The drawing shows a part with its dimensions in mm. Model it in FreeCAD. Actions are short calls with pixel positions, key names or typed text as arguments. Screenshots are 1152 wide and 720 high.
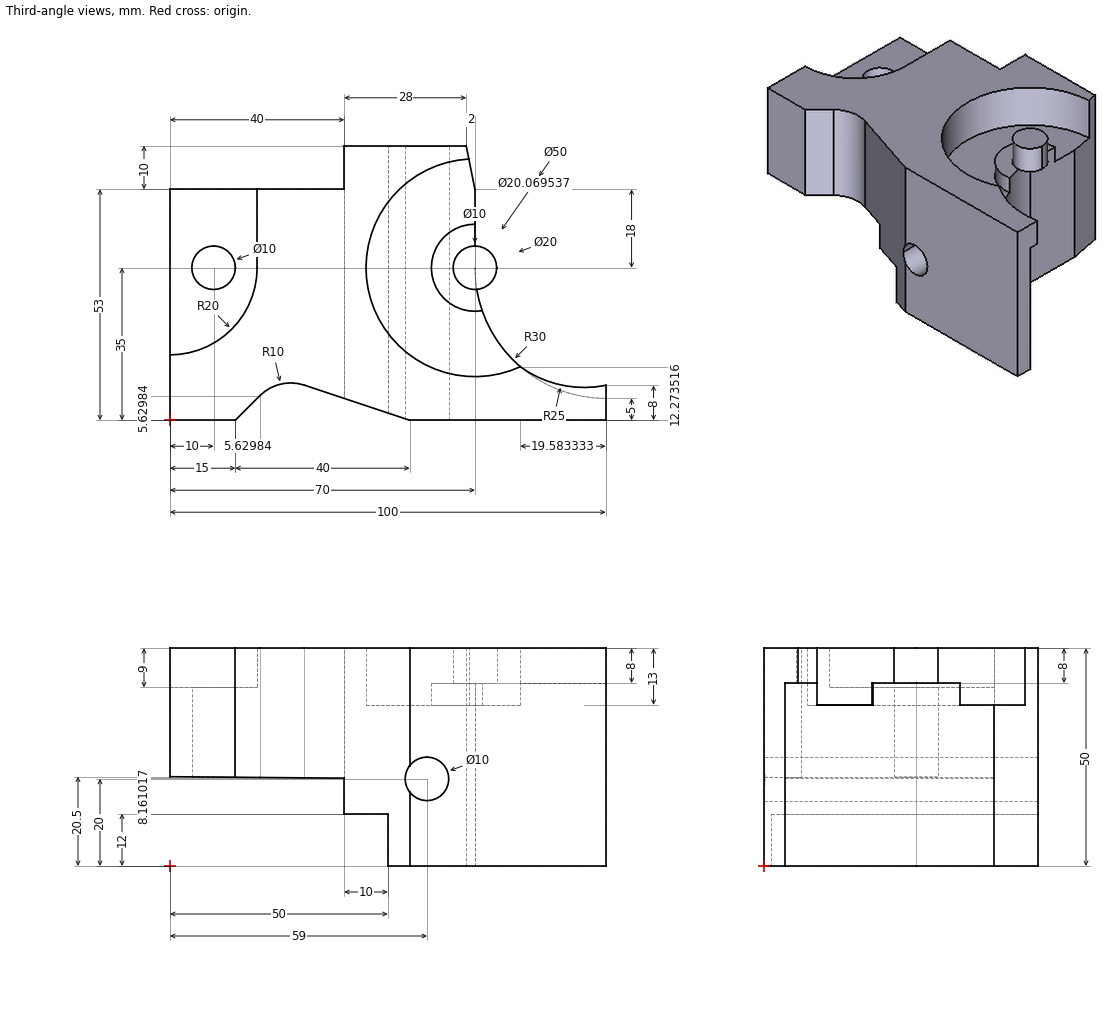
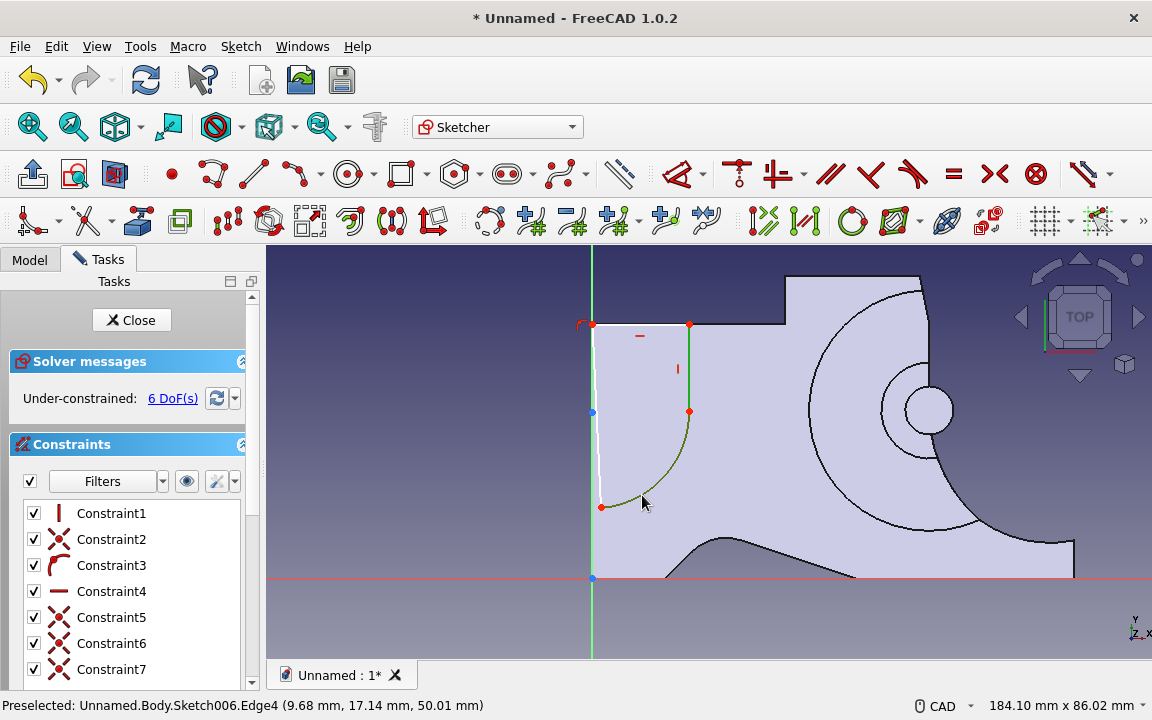
click(913, 174)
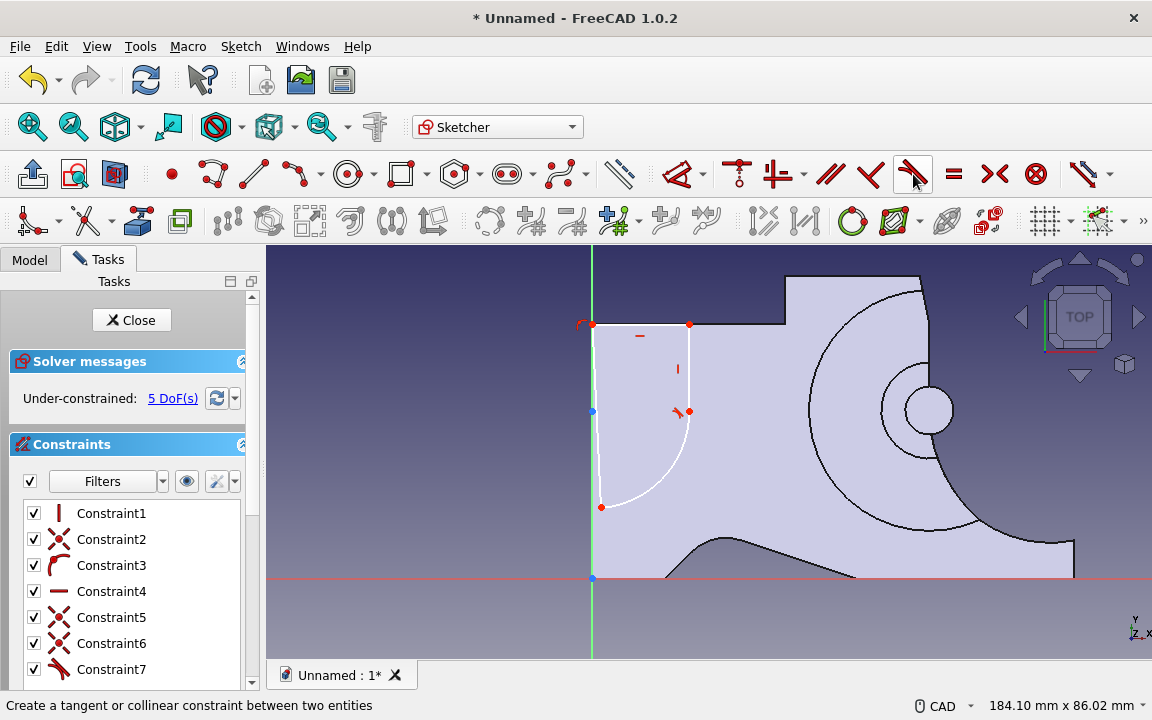
click(595, 380)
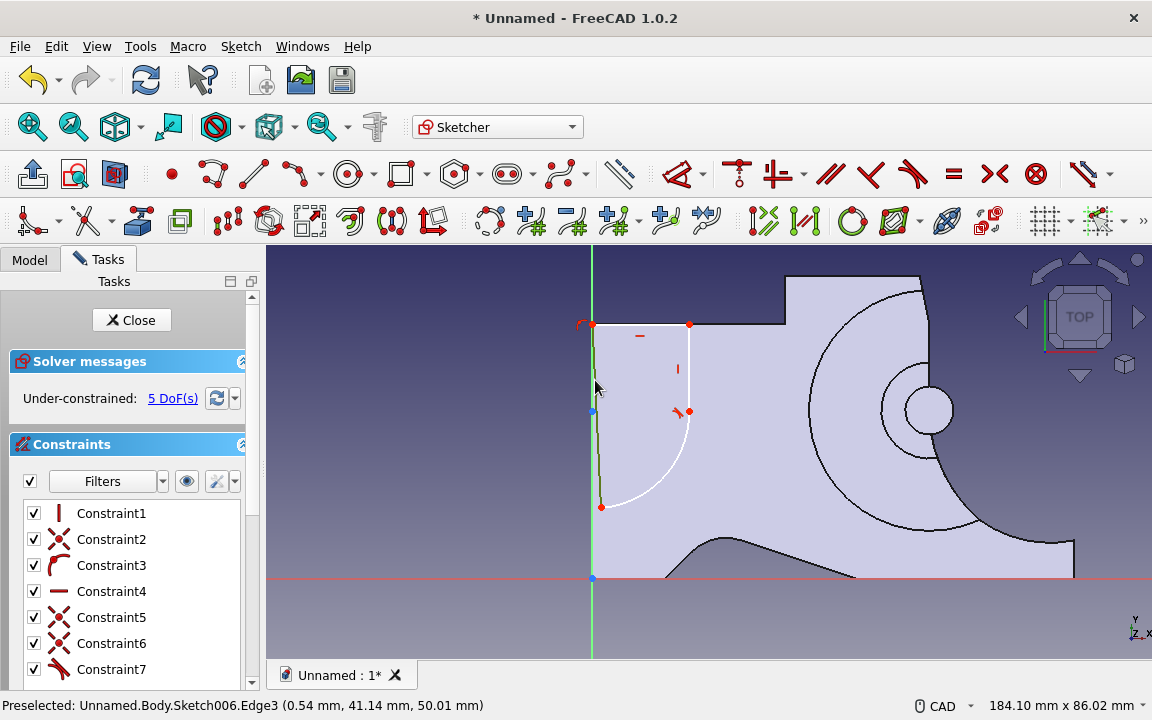
key(v)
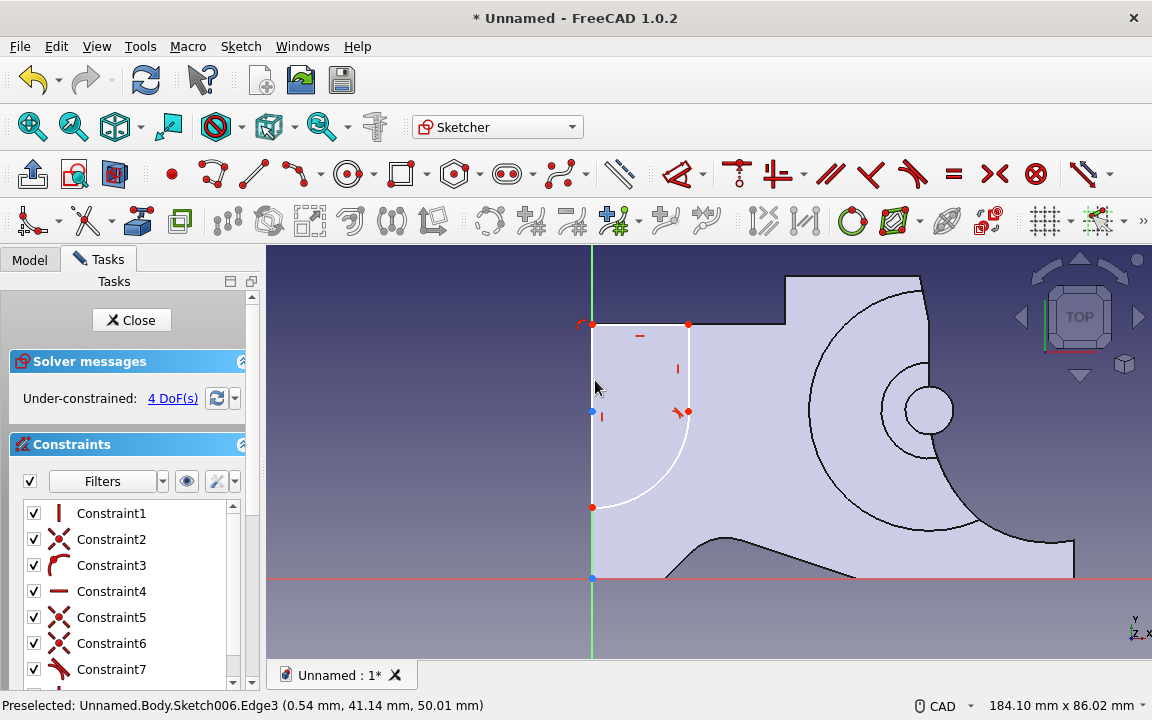
click(593, 412)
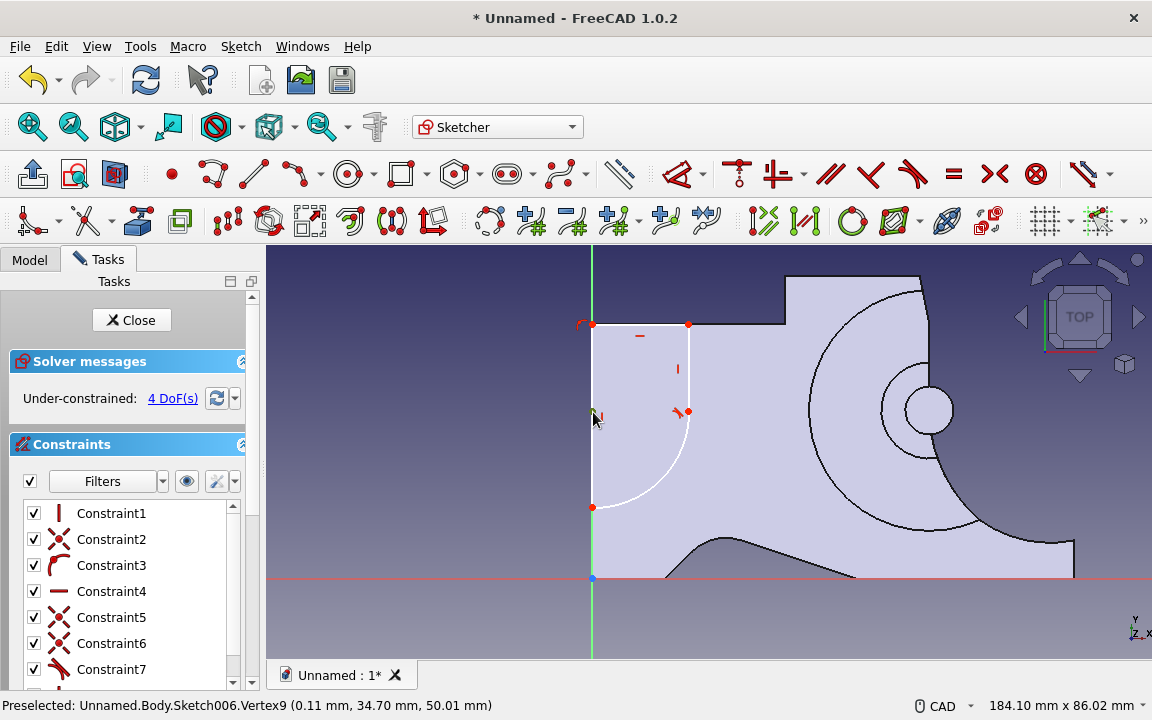
click(592, 605)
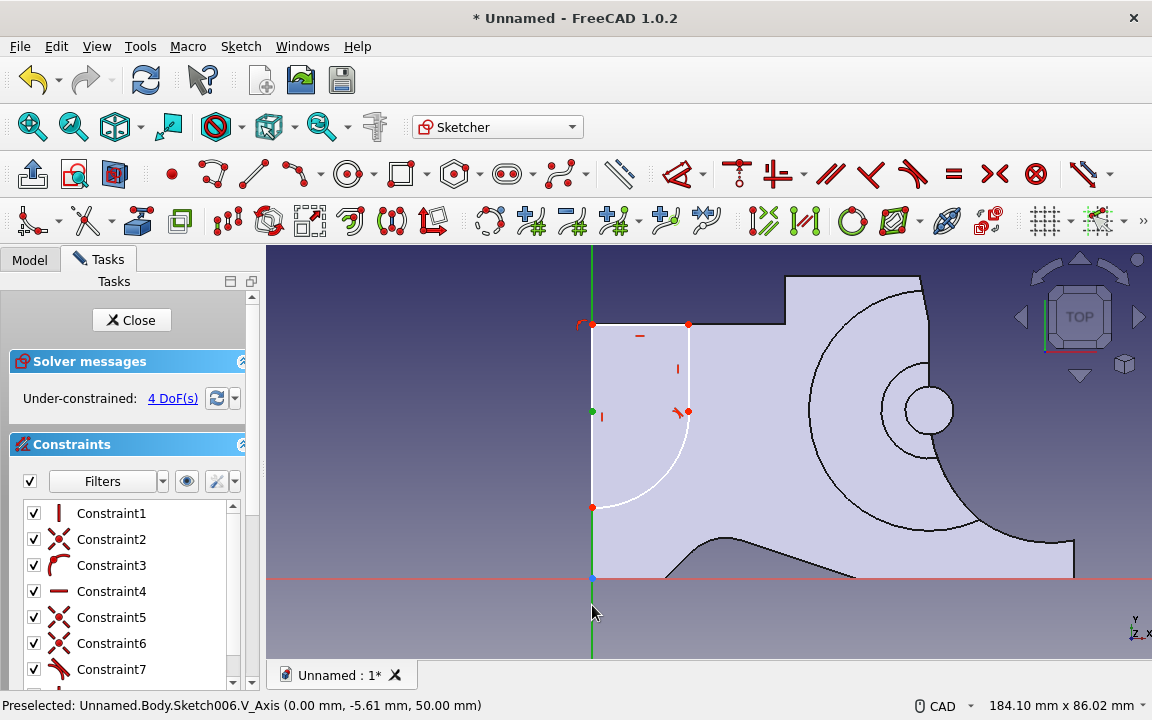
click(737, 174)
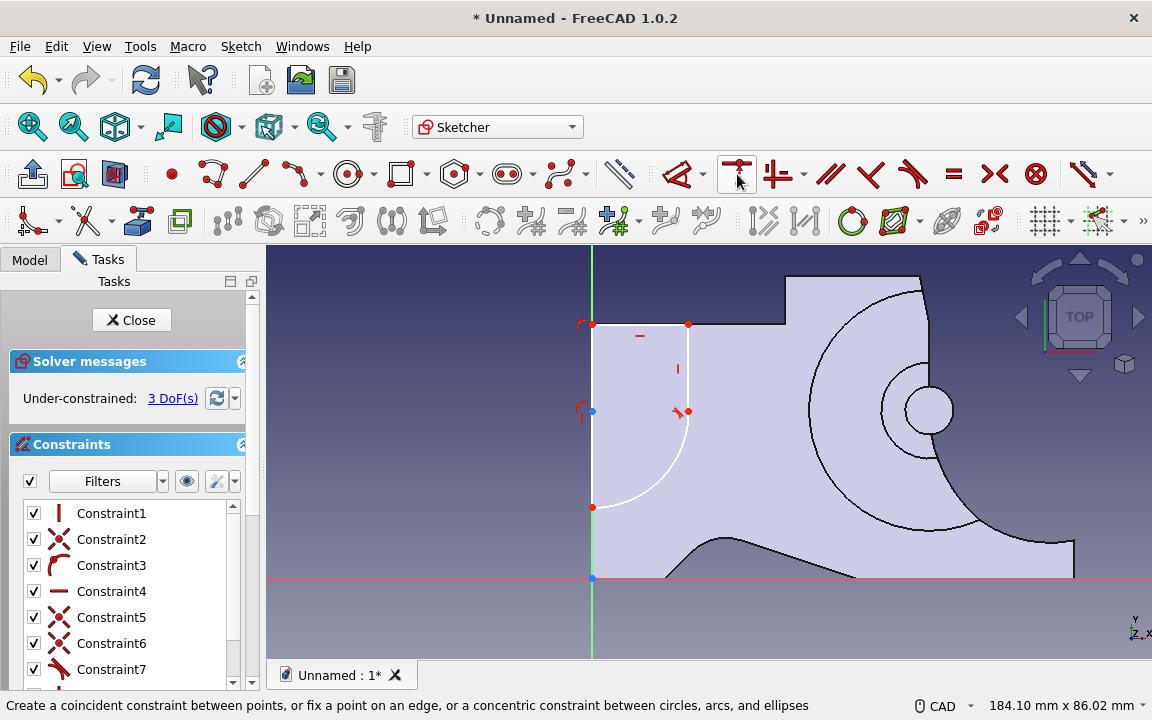
key(d)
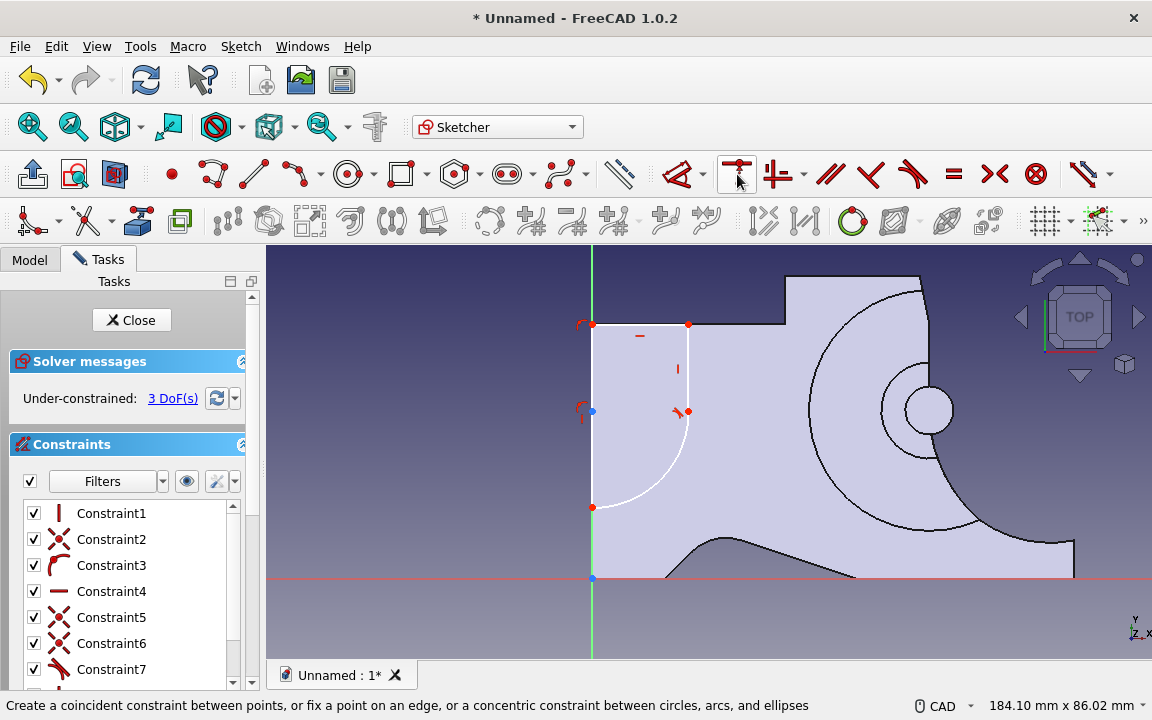
click(636, 498)
click(650, 527)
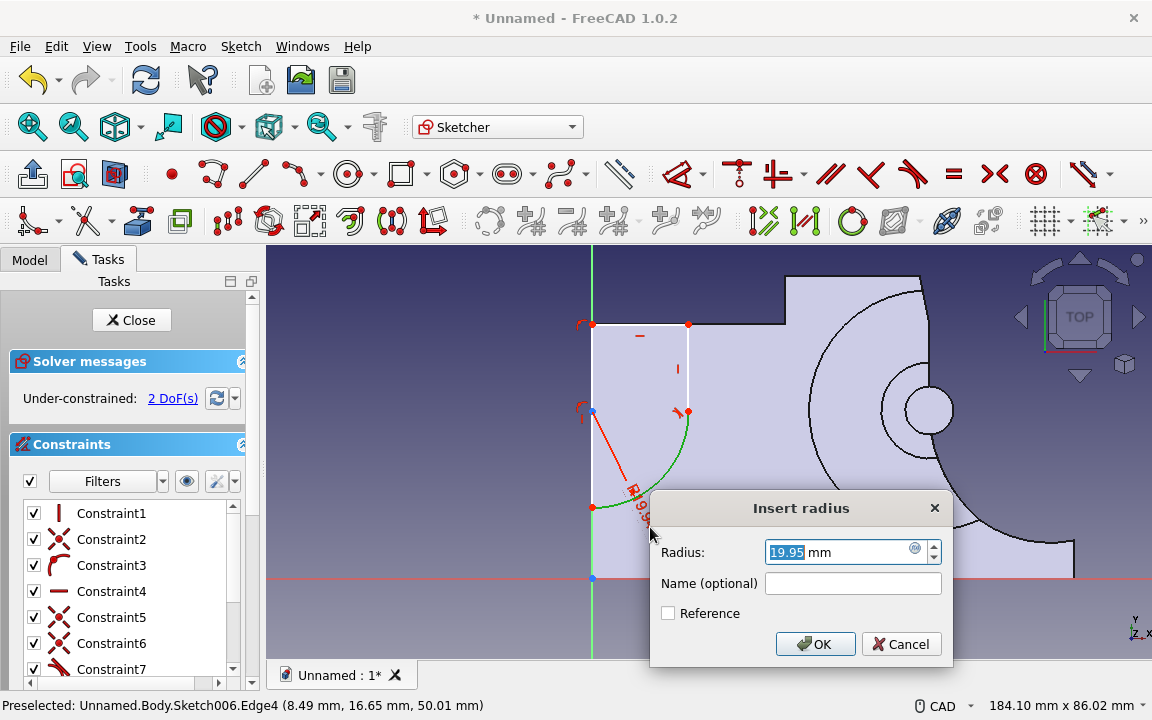
text(20)
key(Return)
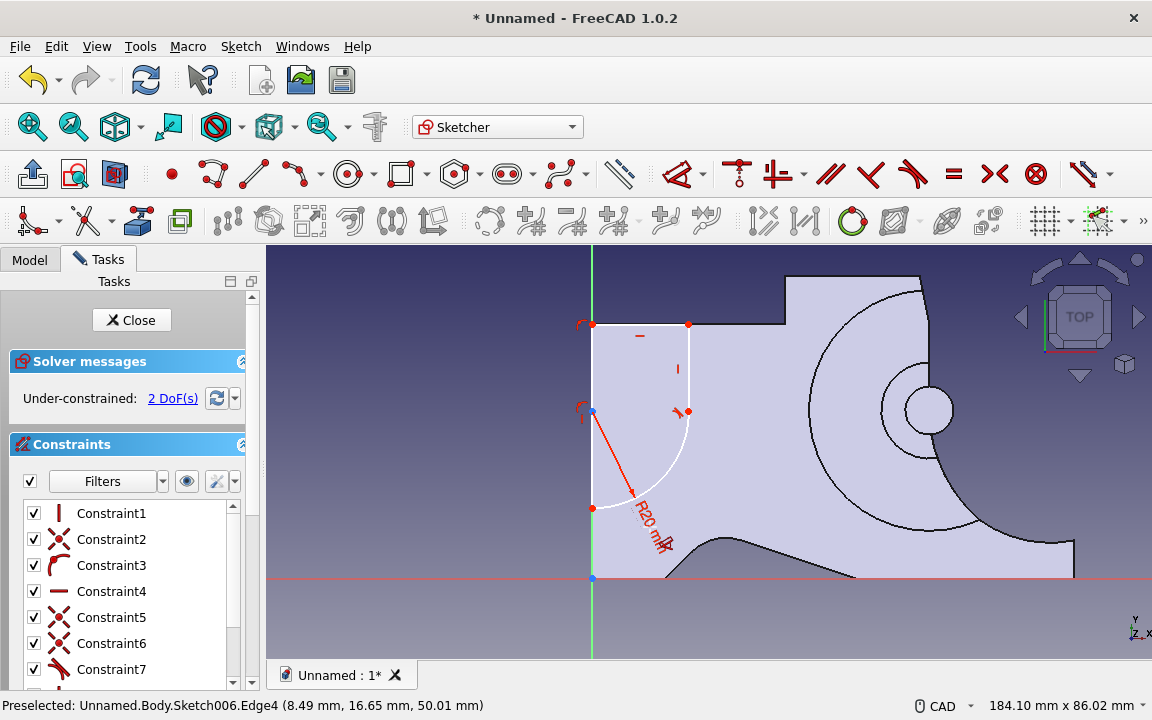
click(689, 386)
click(723, 369)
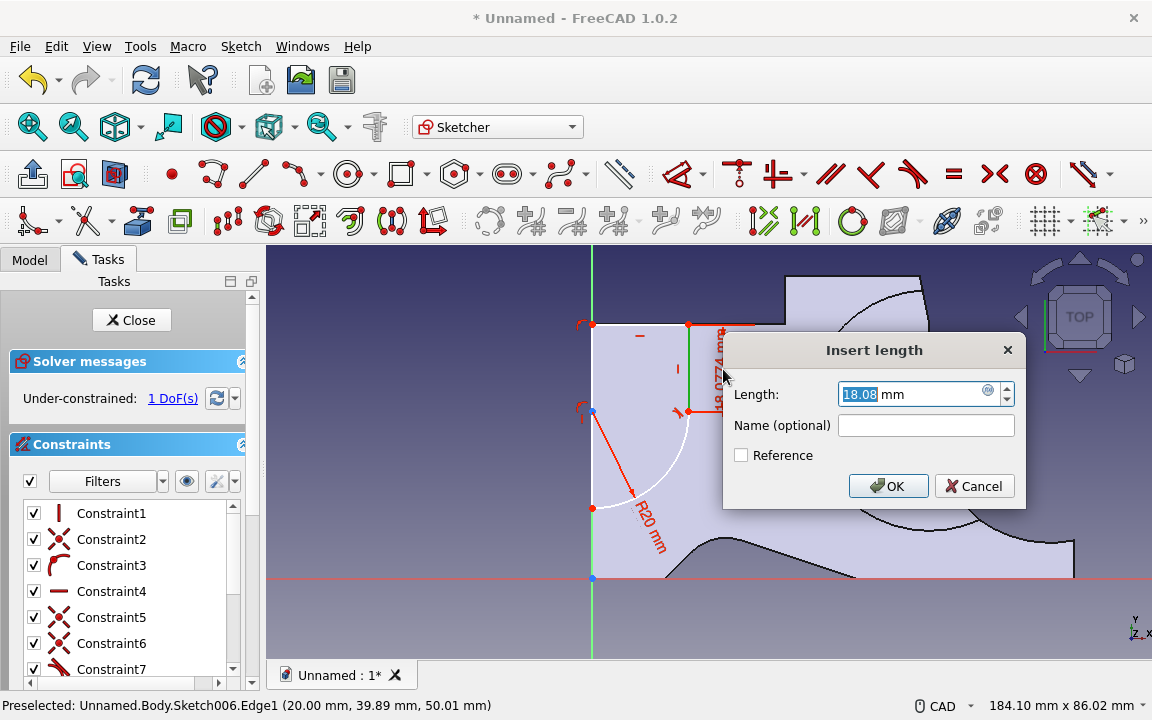
text(18)
key(Return)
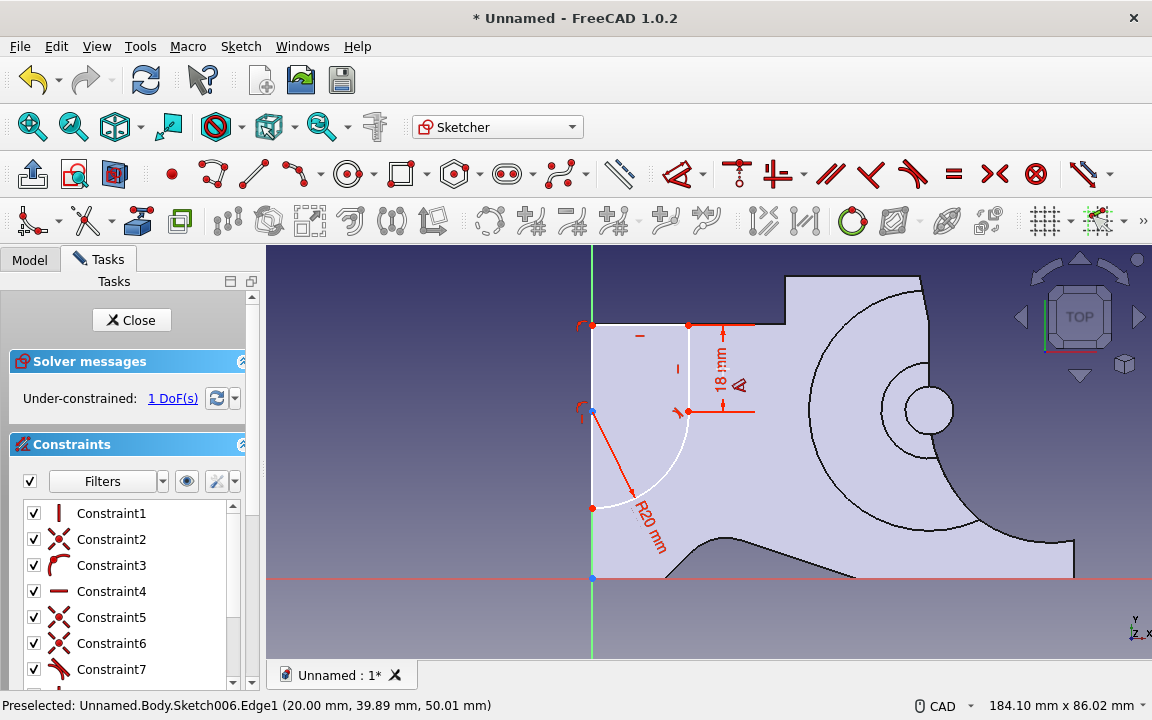
click(689, 412)
click(723, 495)